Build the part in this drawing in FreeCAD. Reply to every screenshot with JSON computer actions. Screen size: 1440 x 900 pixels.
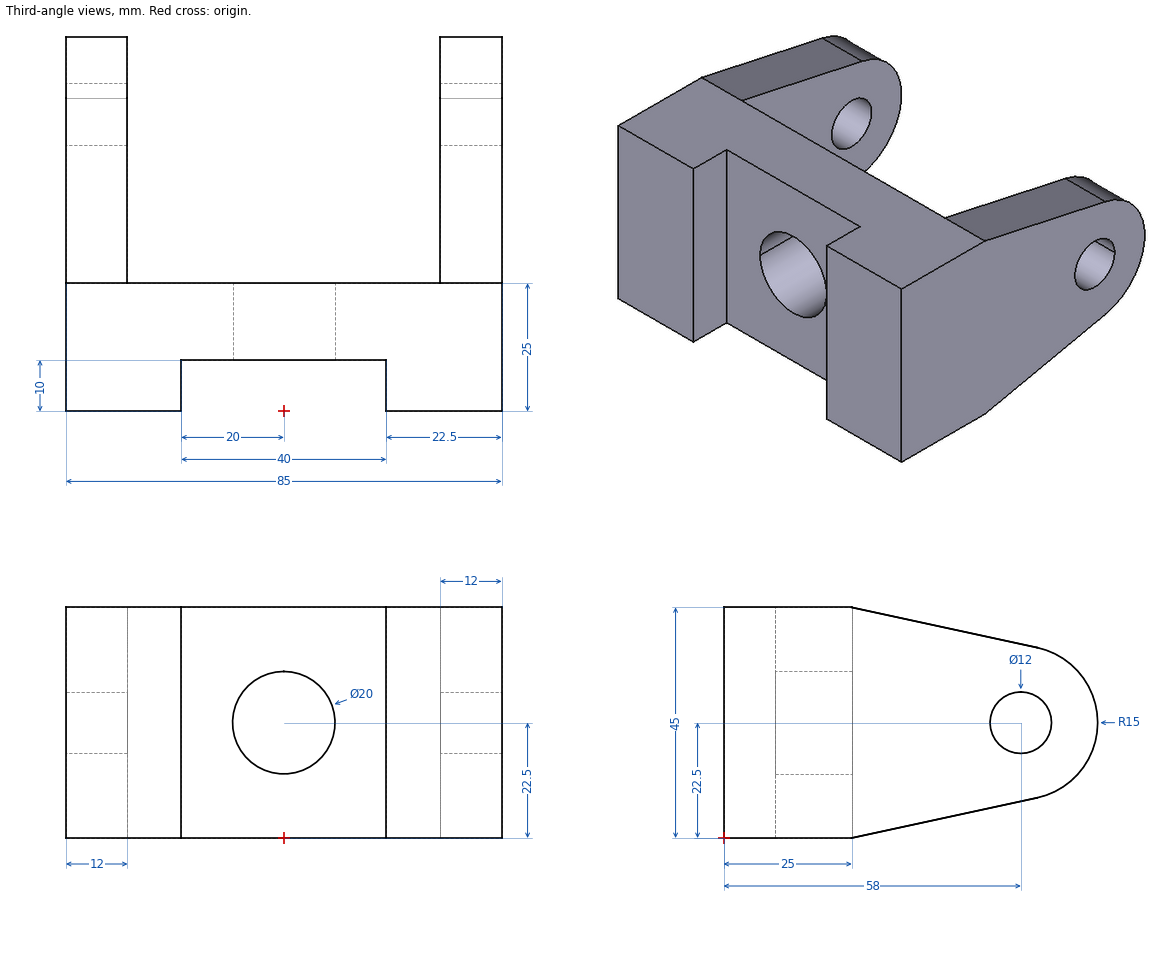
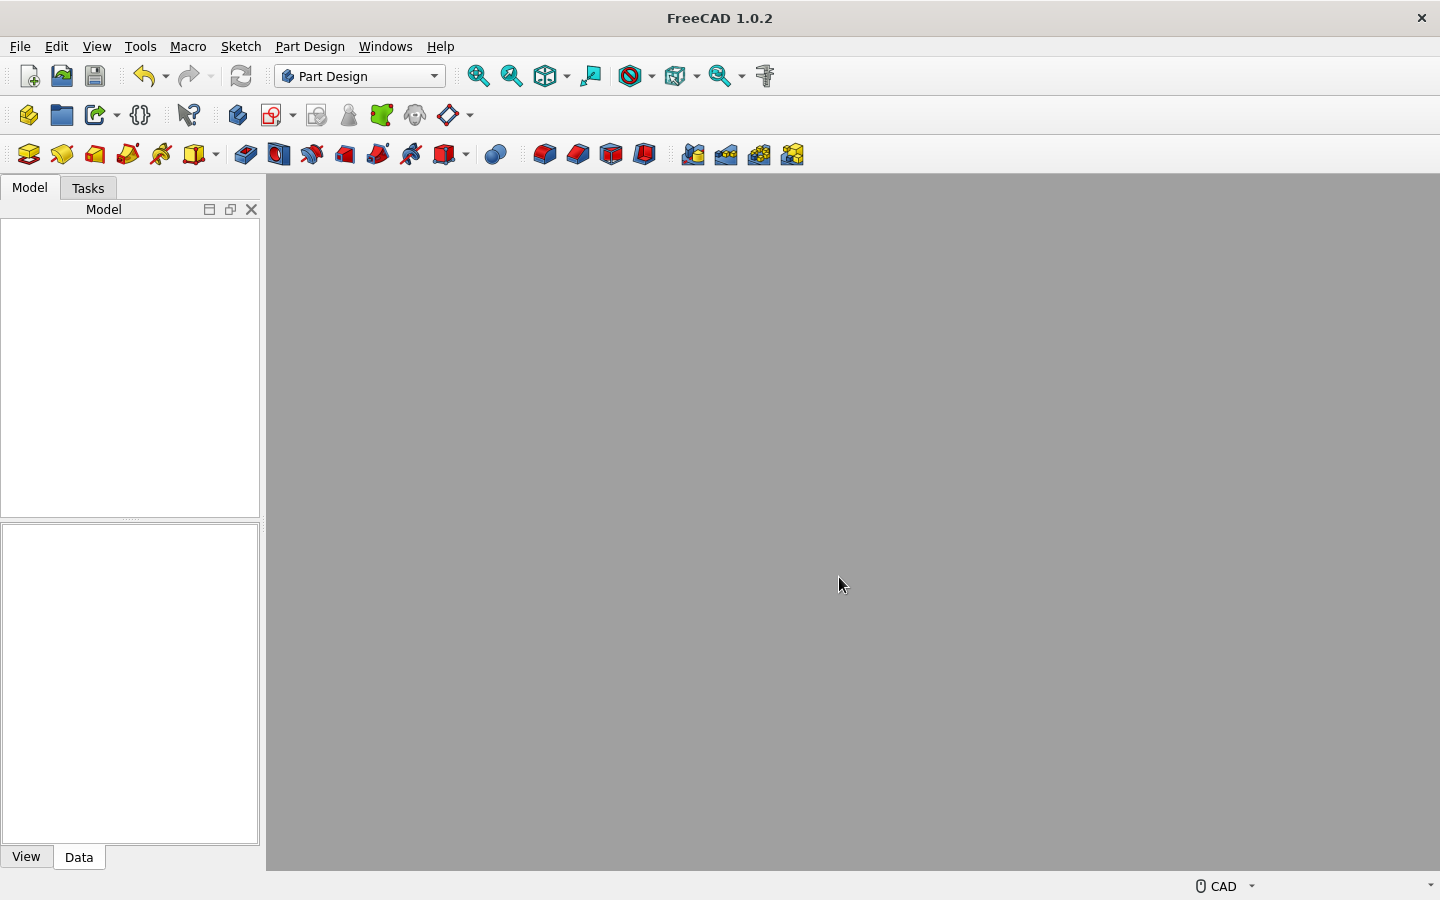
{"action": "left_click", "coordinate": [29, 76]}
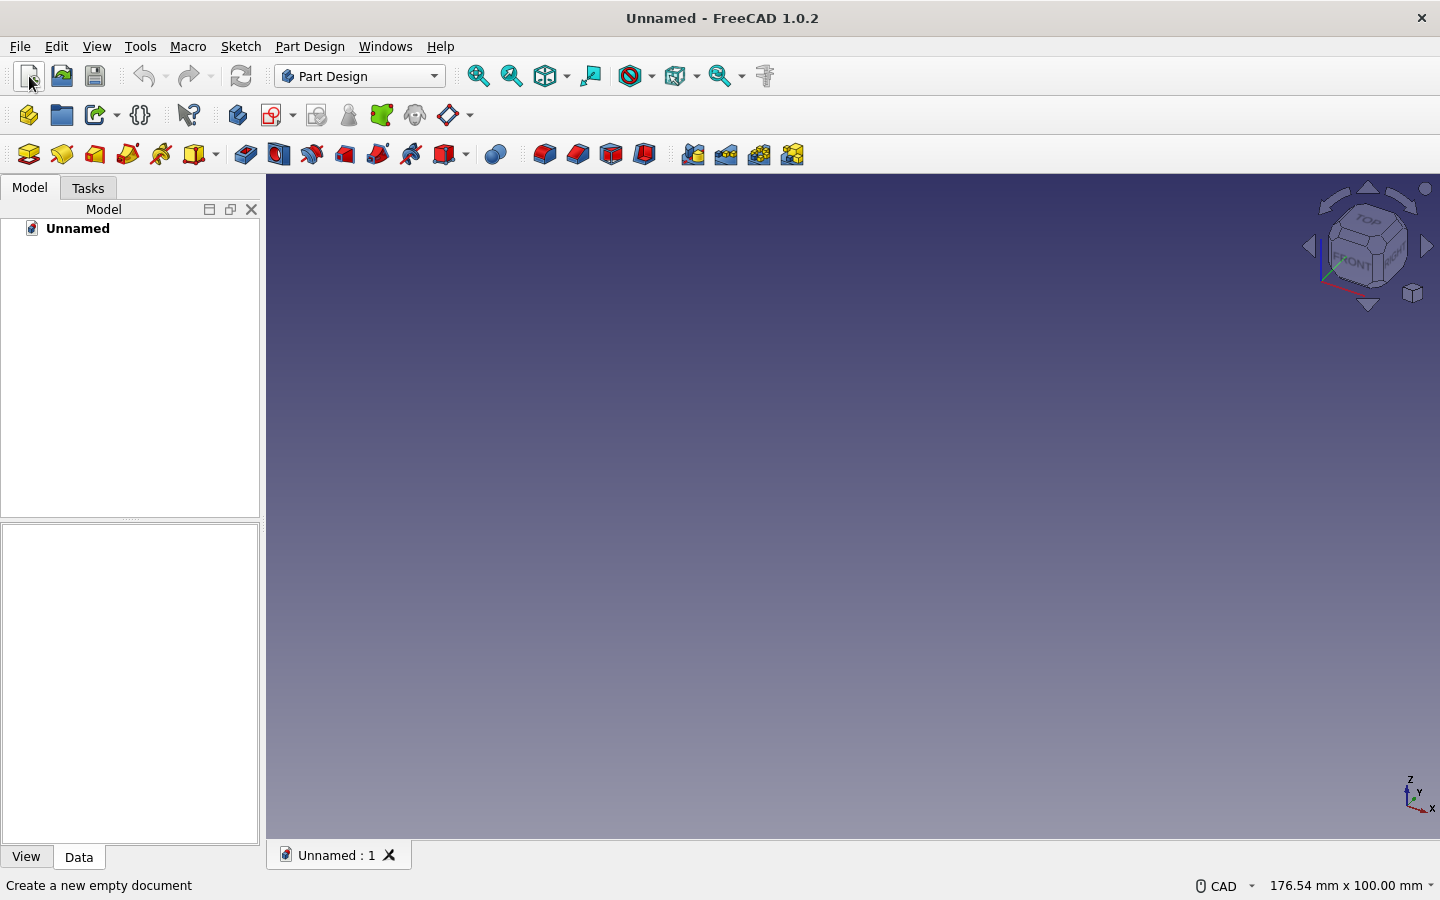
{"action": "left_click", "coordinate": [270, 116]}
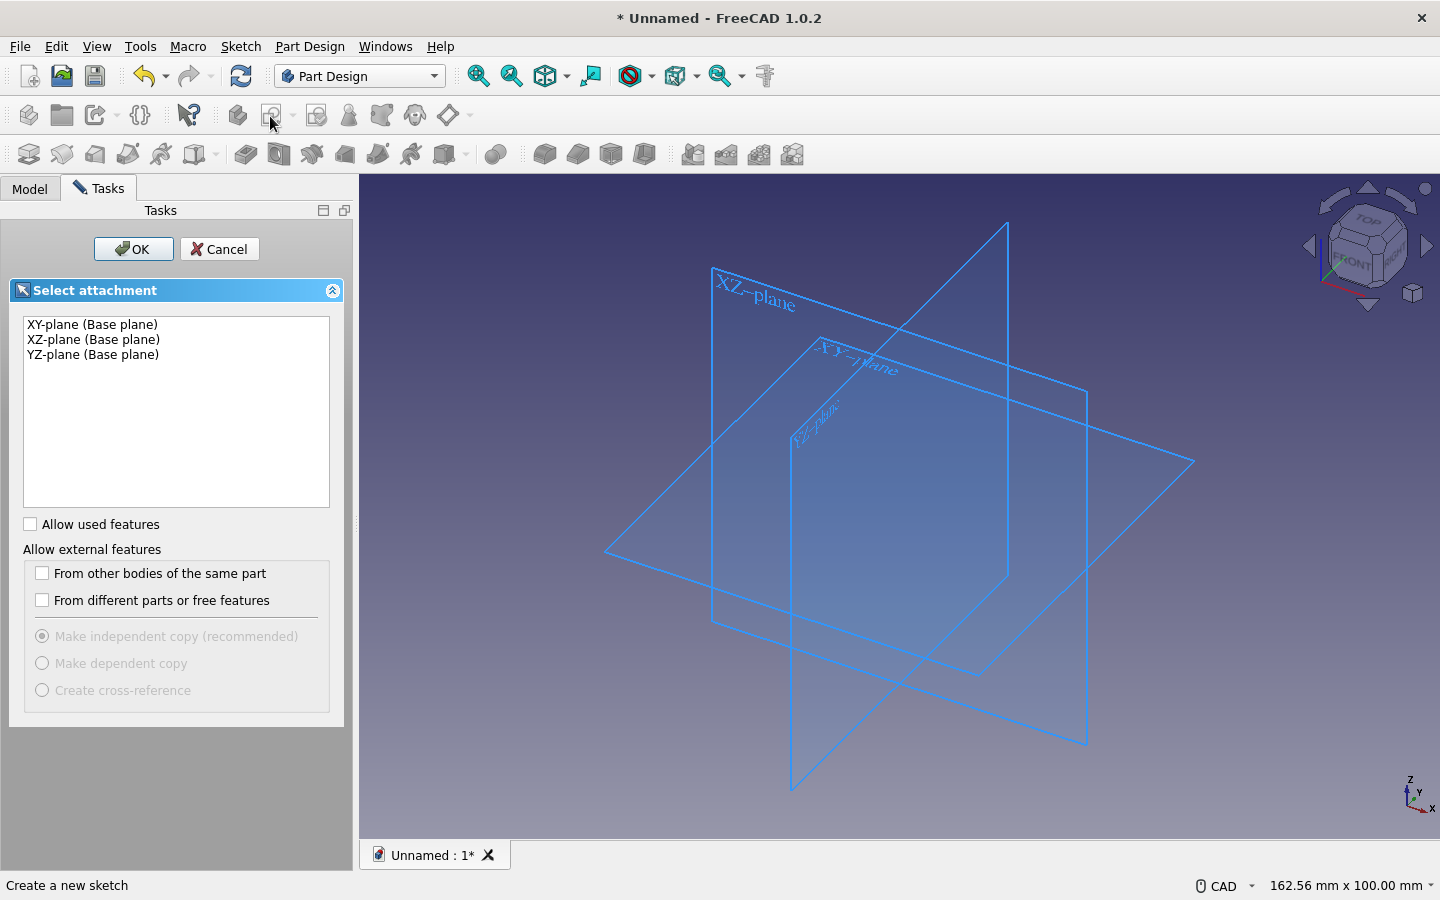
{"action": "left_click", "coordinate": [84, 324]}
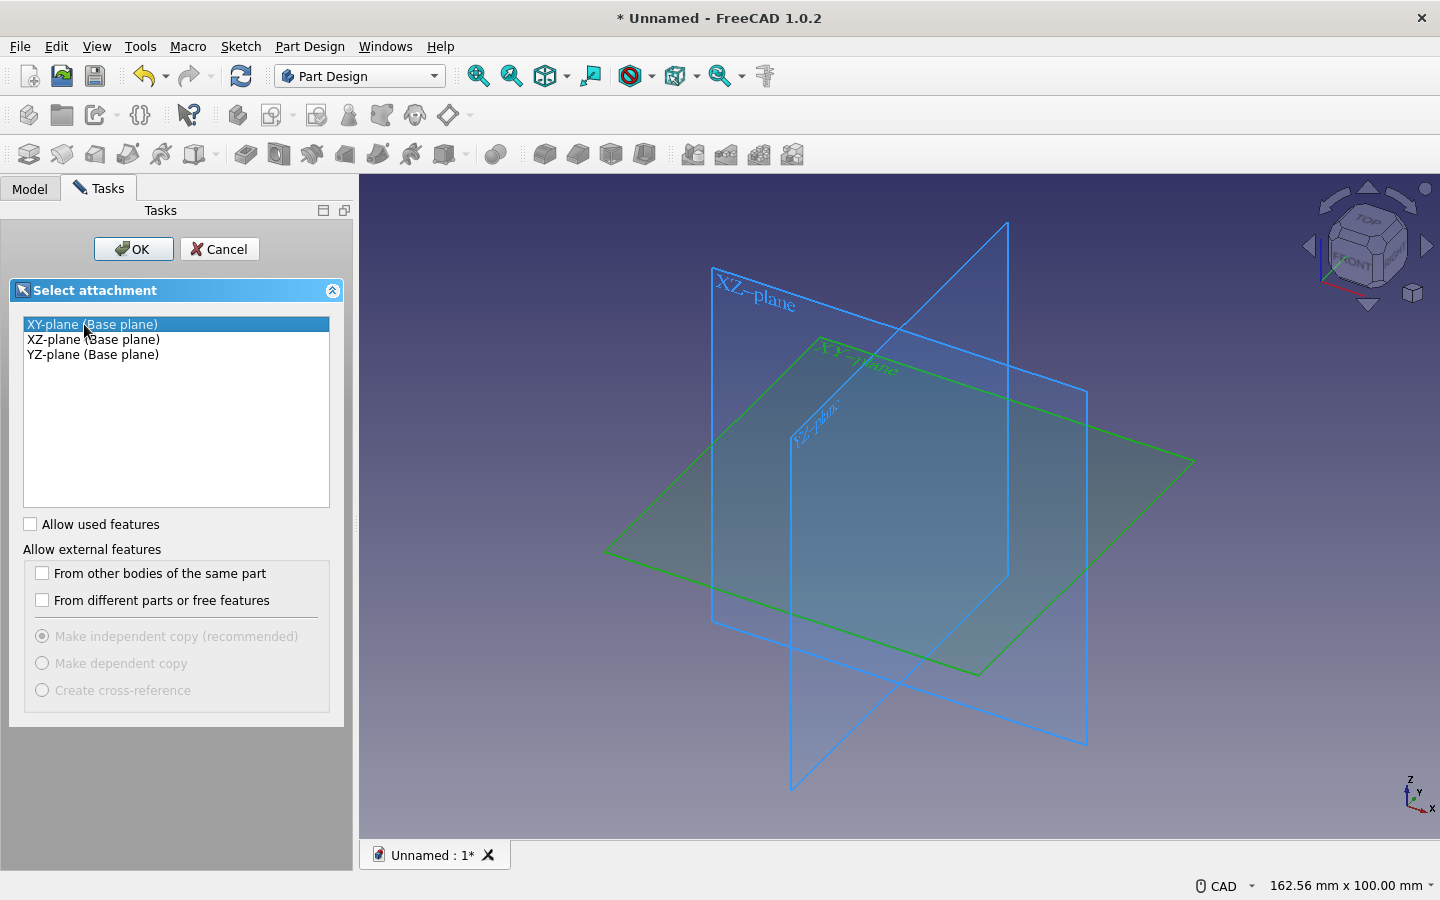
{"action": "left_click", "coordinate": [134, 249]}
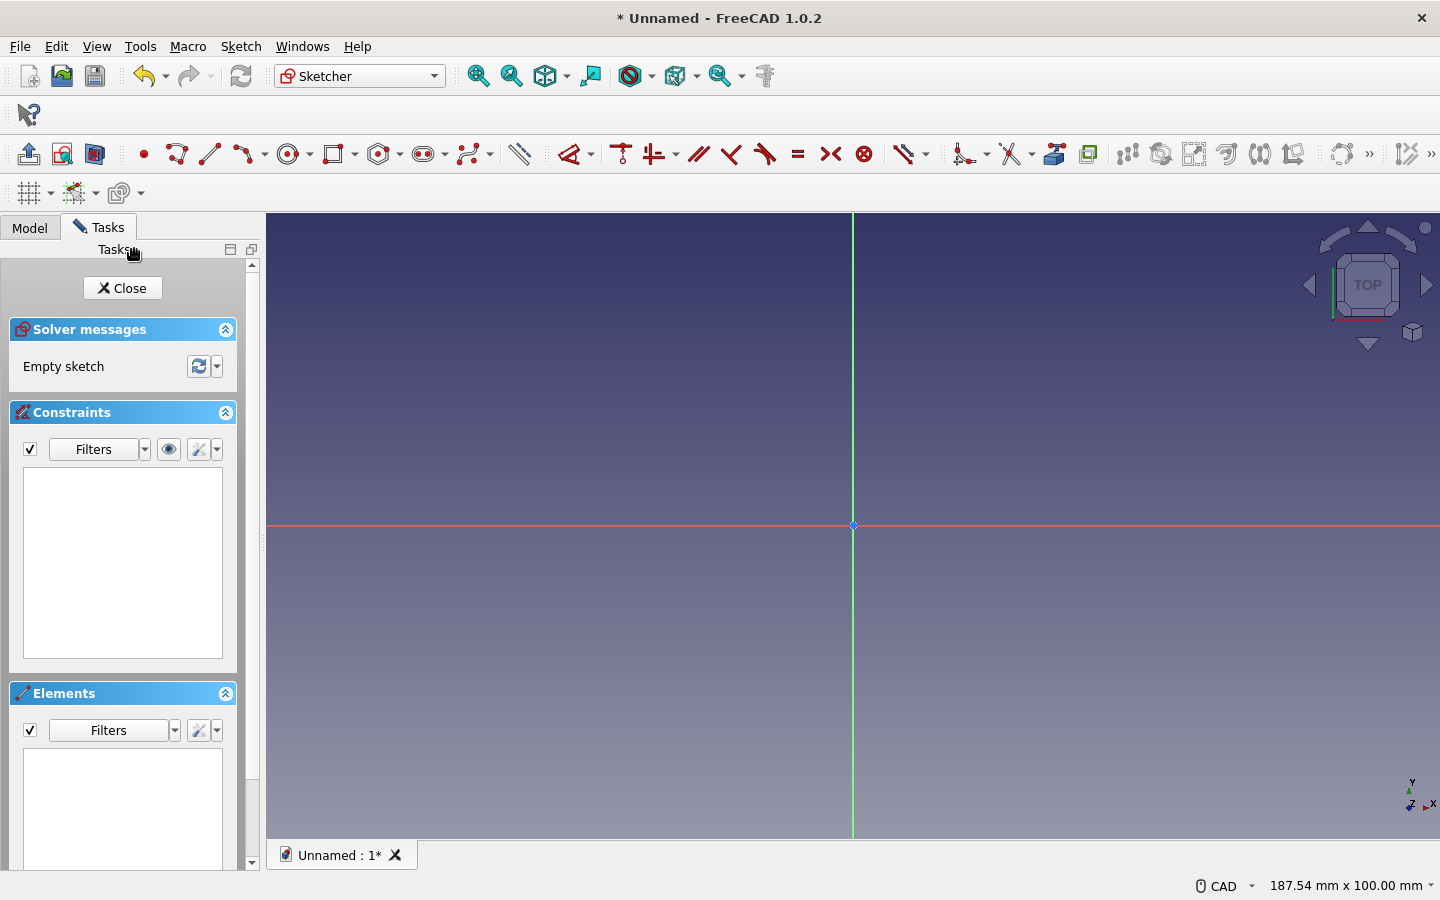
{"action": "left_click", "coordinate": [177, 154]}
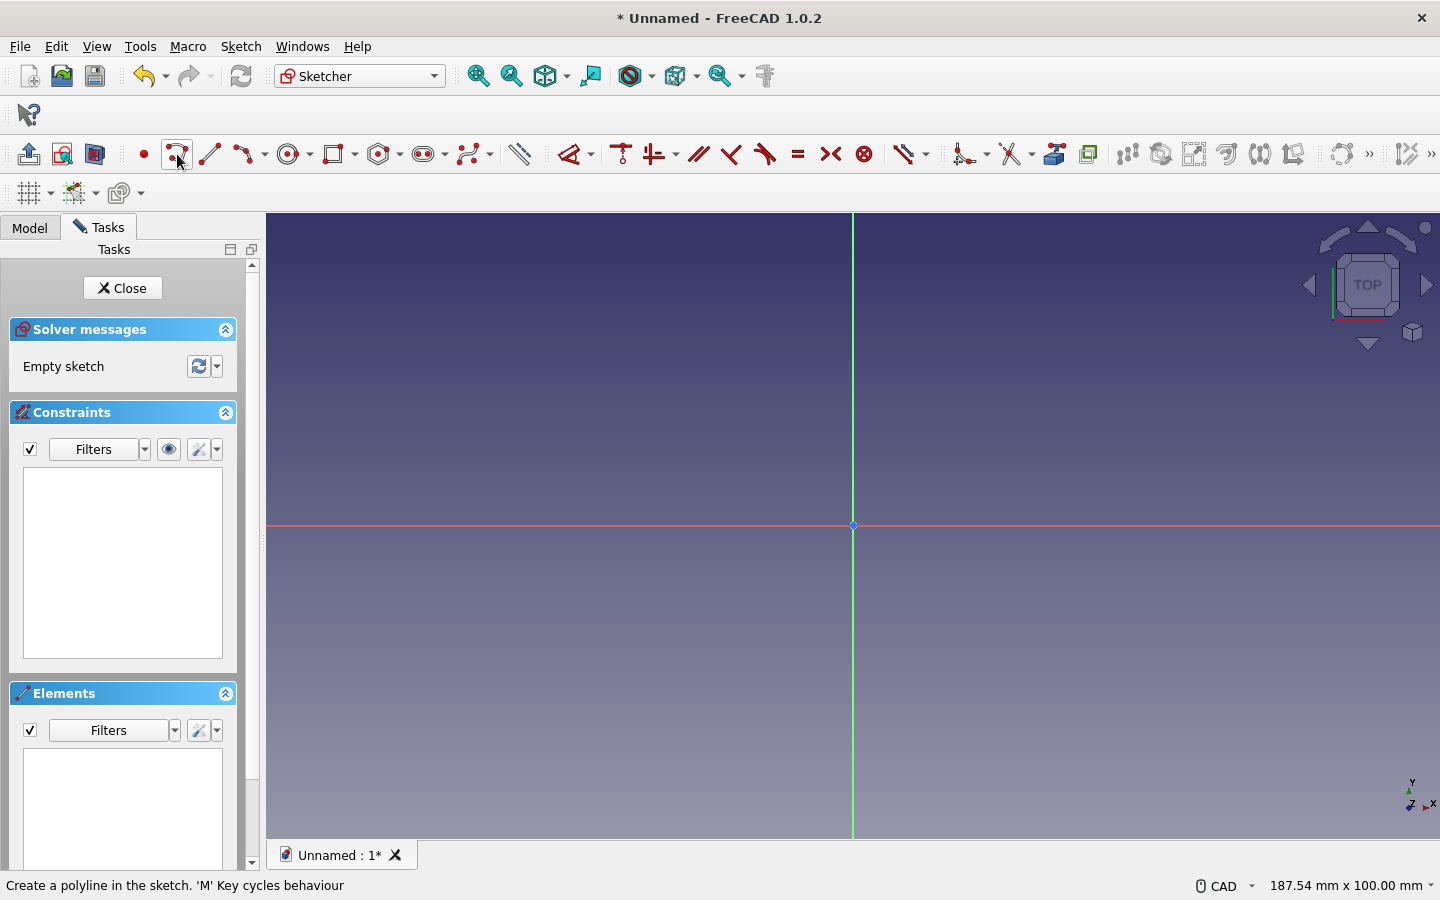
{"action": "left_click", "coordinate": [728, 526]}
{"action": "left_click", "coordinate": [728, 463]}
{"action": "left_click", "coordinate": [978, 463]}
{"action": "left_click", "coordinate": [978, 526]}
{"action": "left_click", "coordinate": [1119, 517]}
{"action": "left_click", "coordinate": [1119, 370]}
{"action": "left_click", "coordinate": [587, 370]}
{"action": "left_click", "coordinate": [587, 517]}
{"action": "left_click", "coordinate": [728, 526]}
{"action": "key", "text": "Escape"}
{"action": "key", "text": "Escape"}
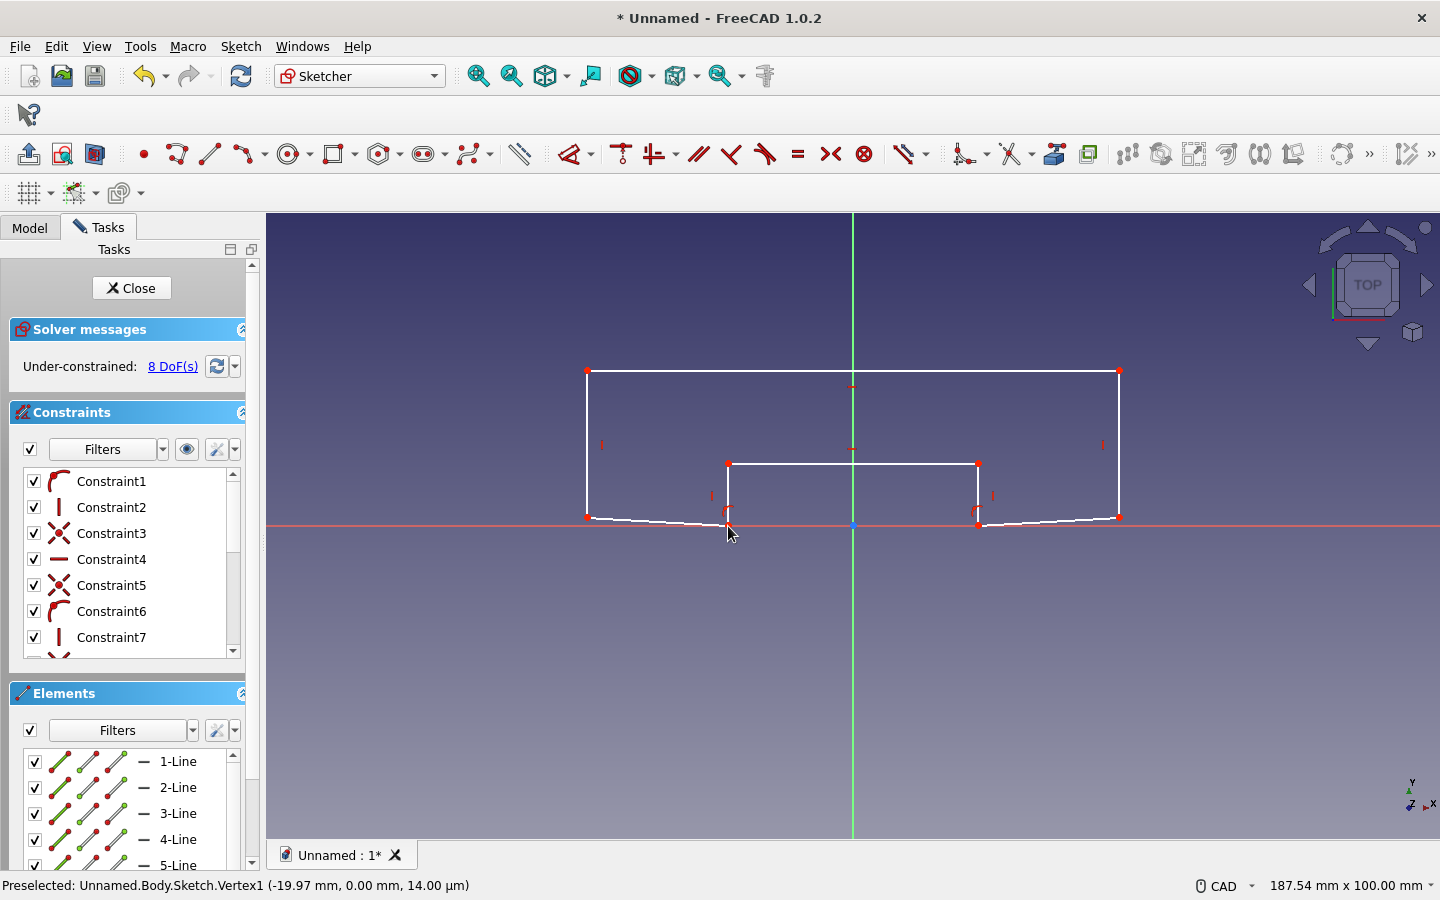
{"action": "left_click", "coordinate": [1020, 524]}